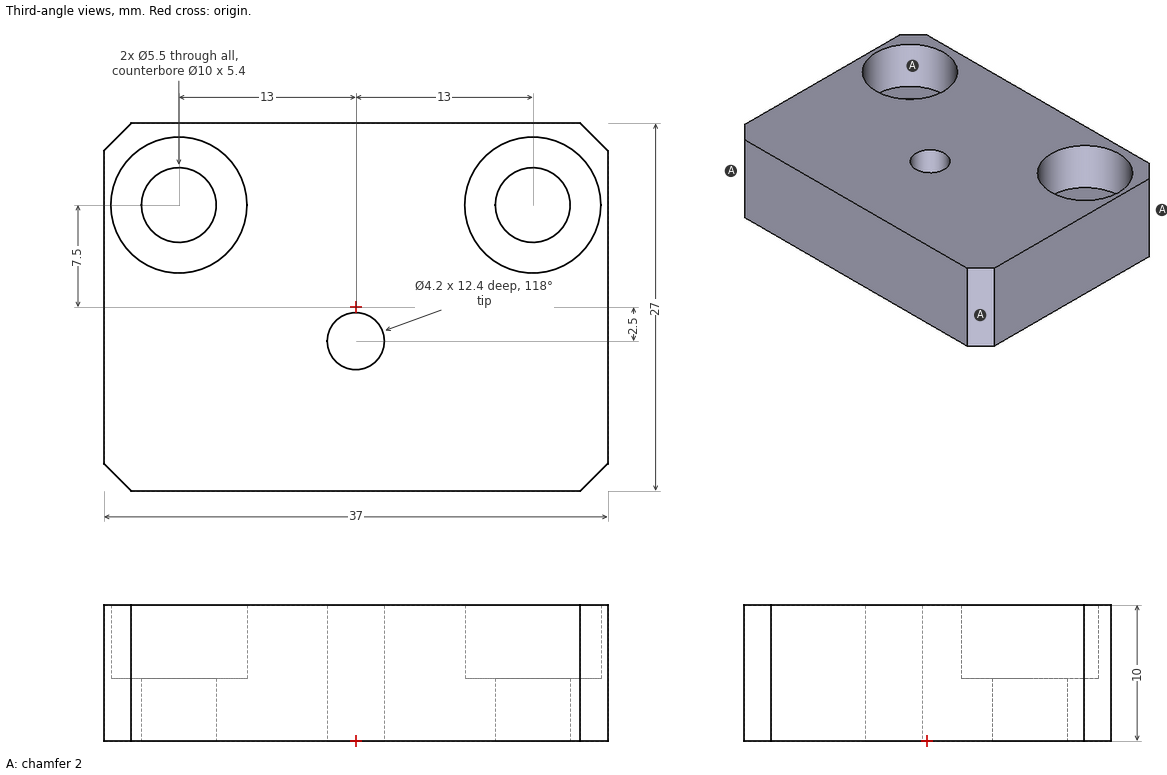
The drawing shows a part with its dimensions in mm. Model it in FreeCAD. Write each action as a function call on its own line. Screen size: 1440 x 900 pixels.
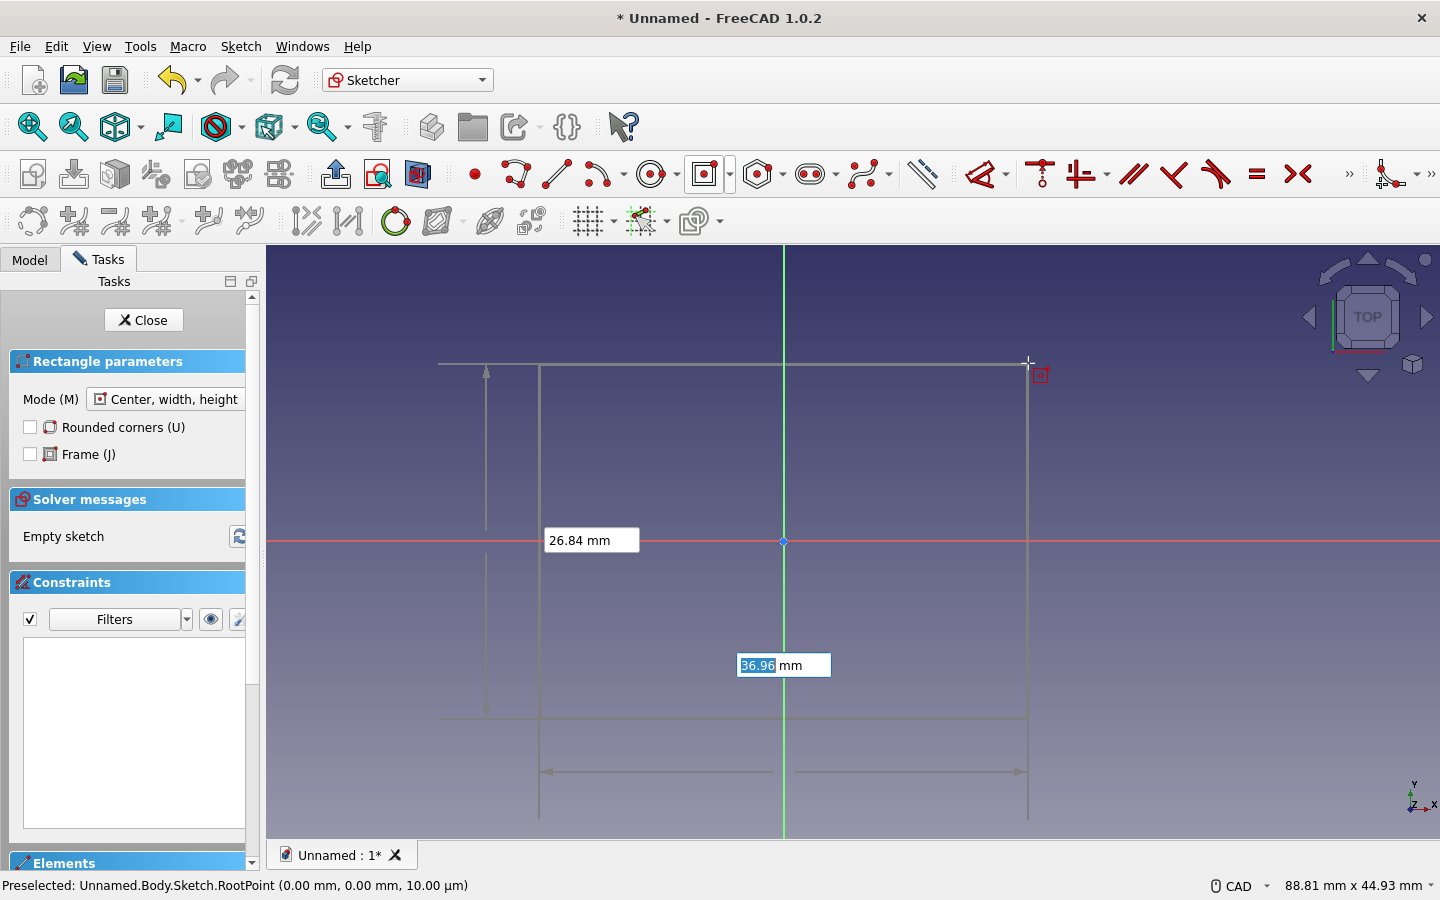
text(37)
key(Tab)
text(27)
key(Return)
key(Escape)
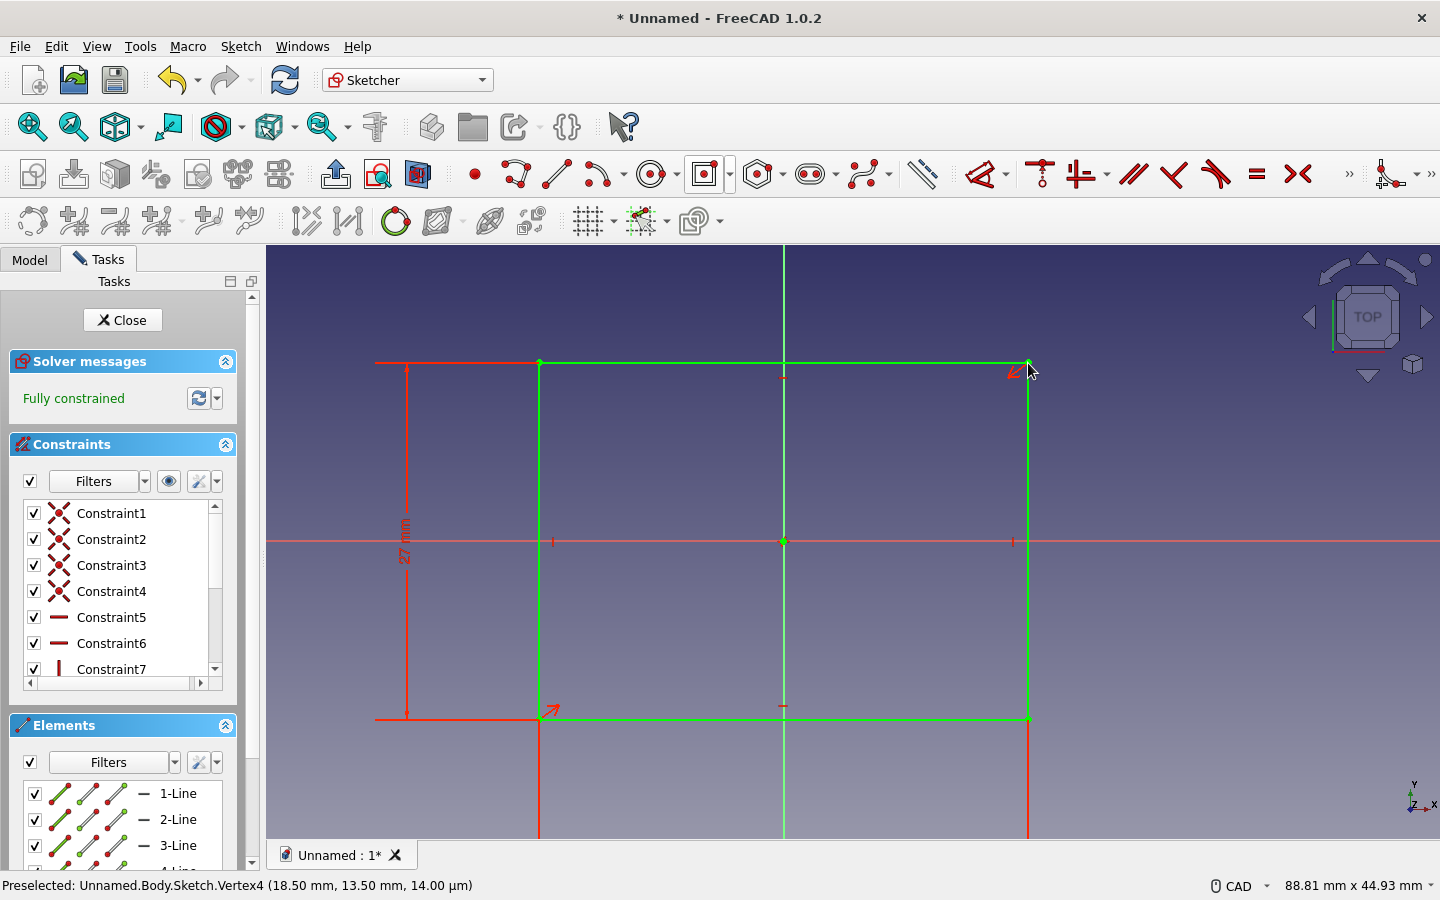
click(123, 320)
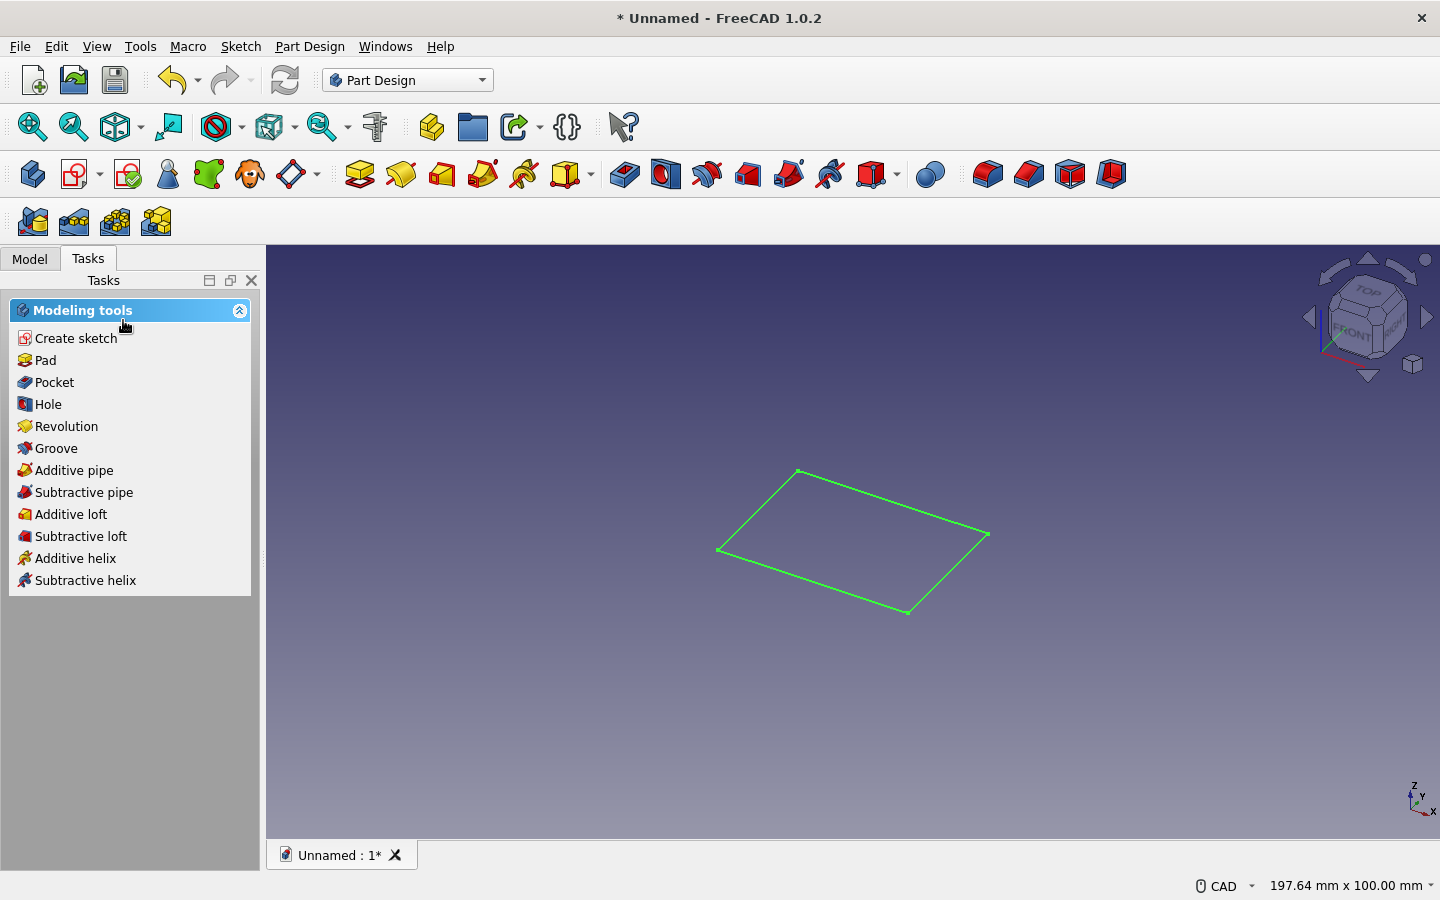
click(360, 174)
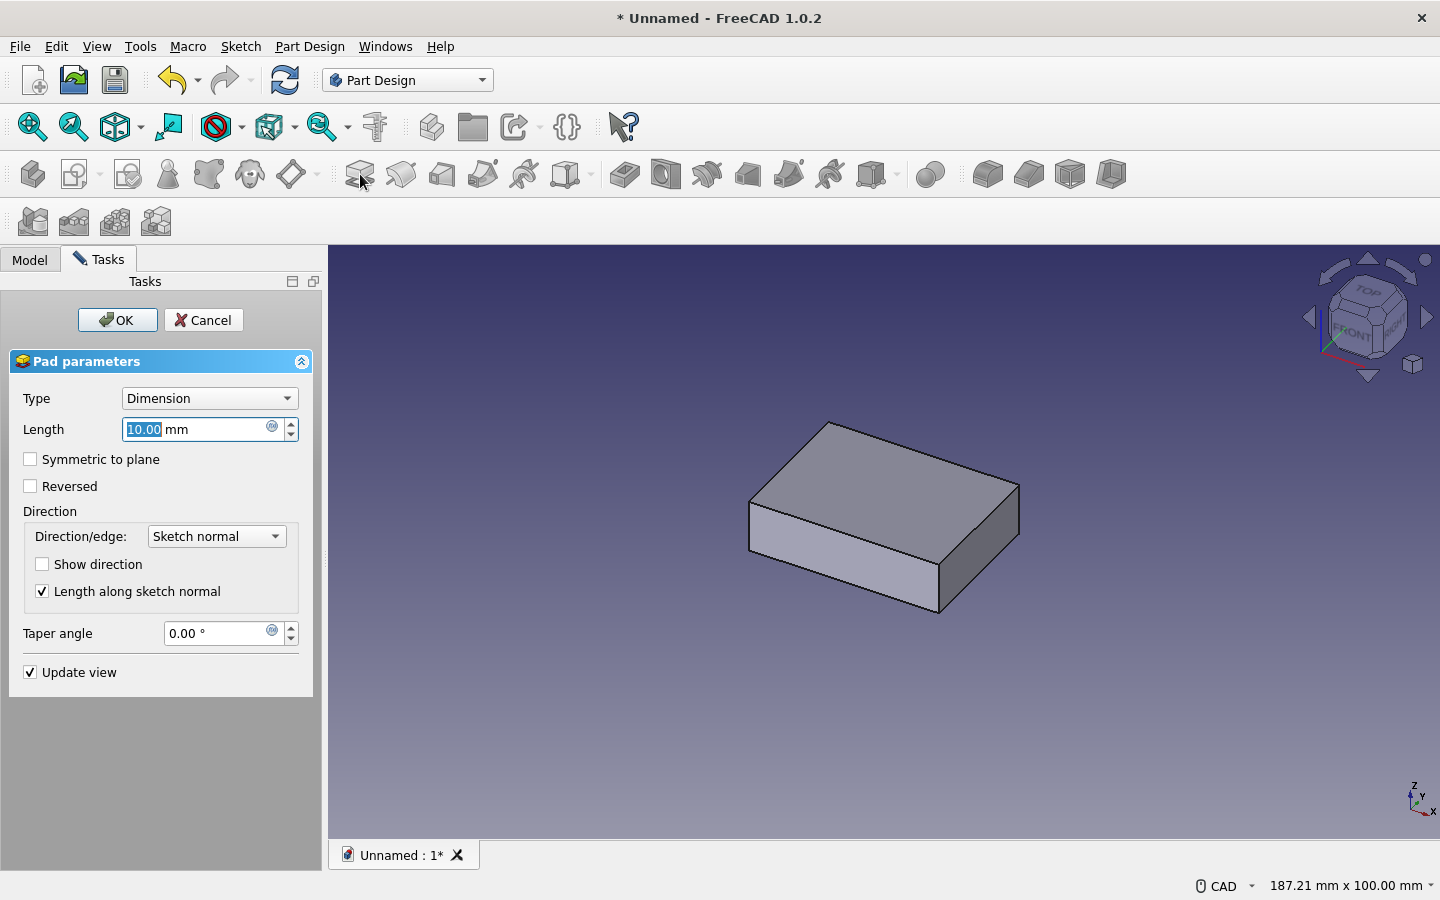
text(10)
key(Tab)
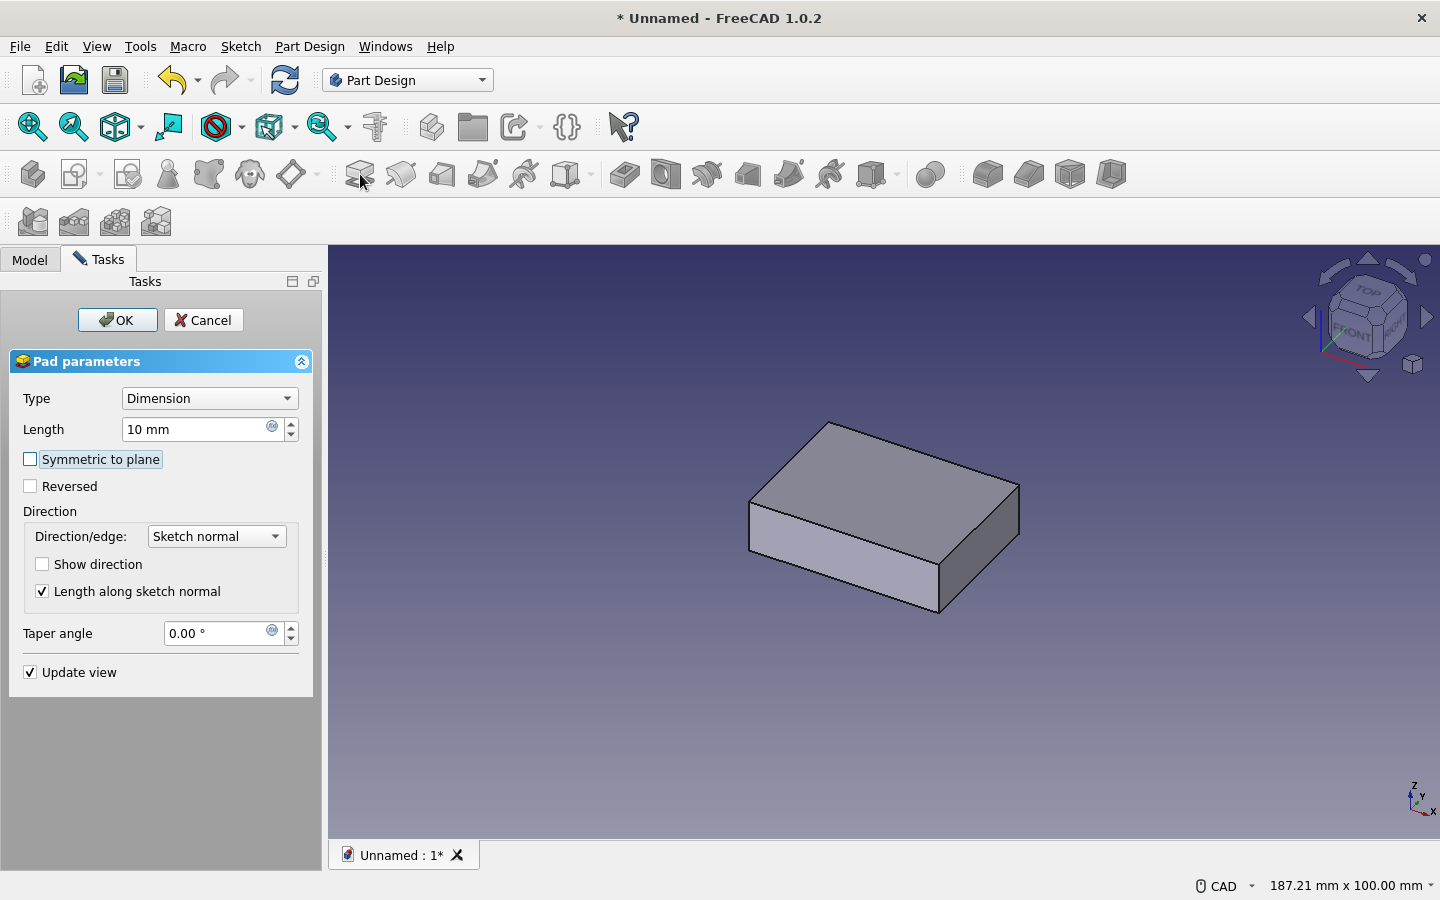
click(118, 320)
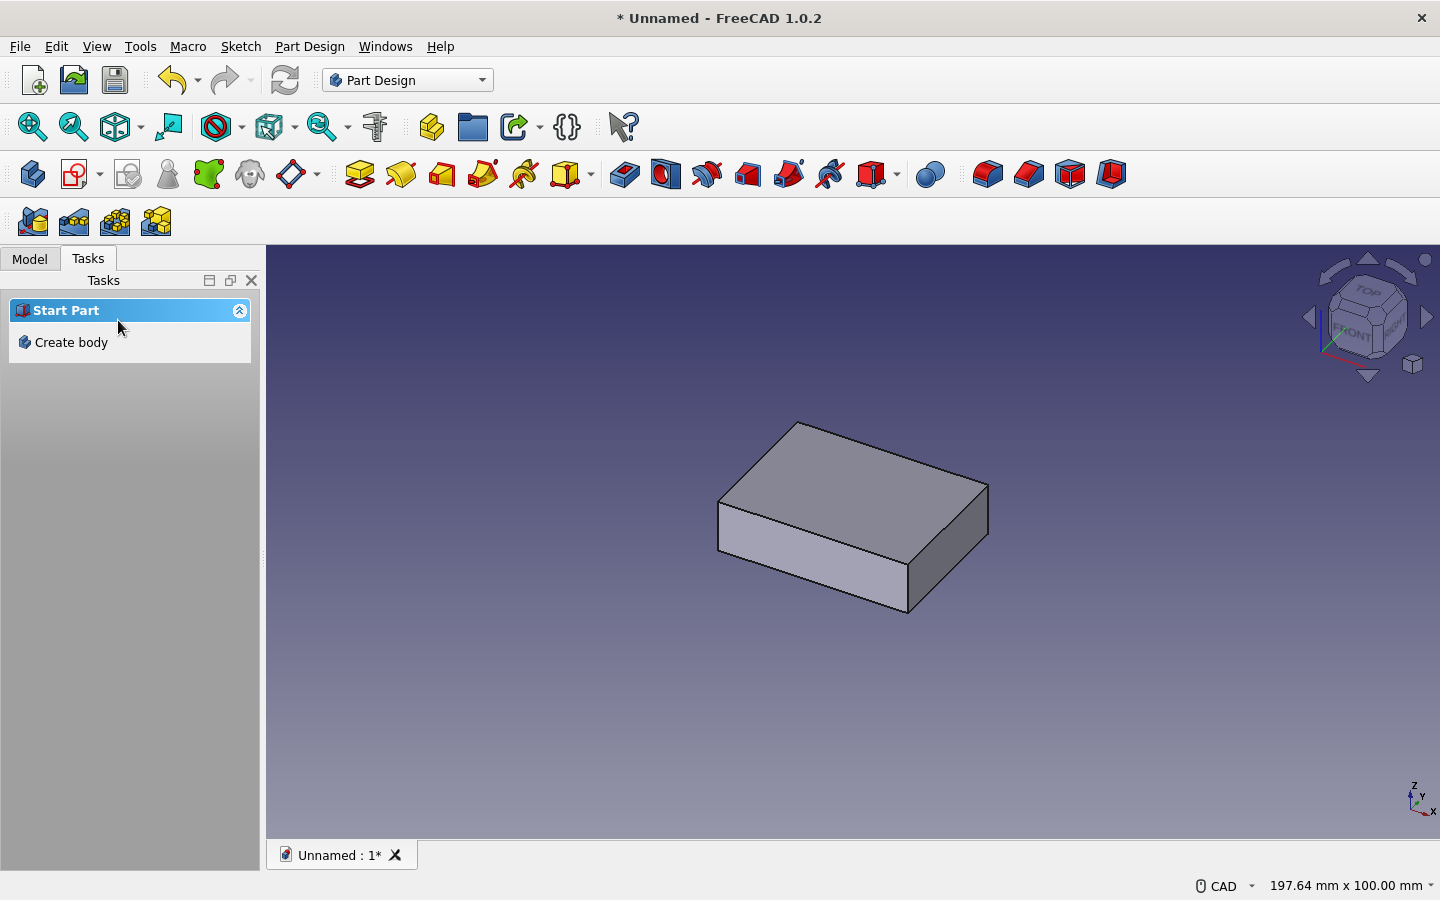
click(33, 128)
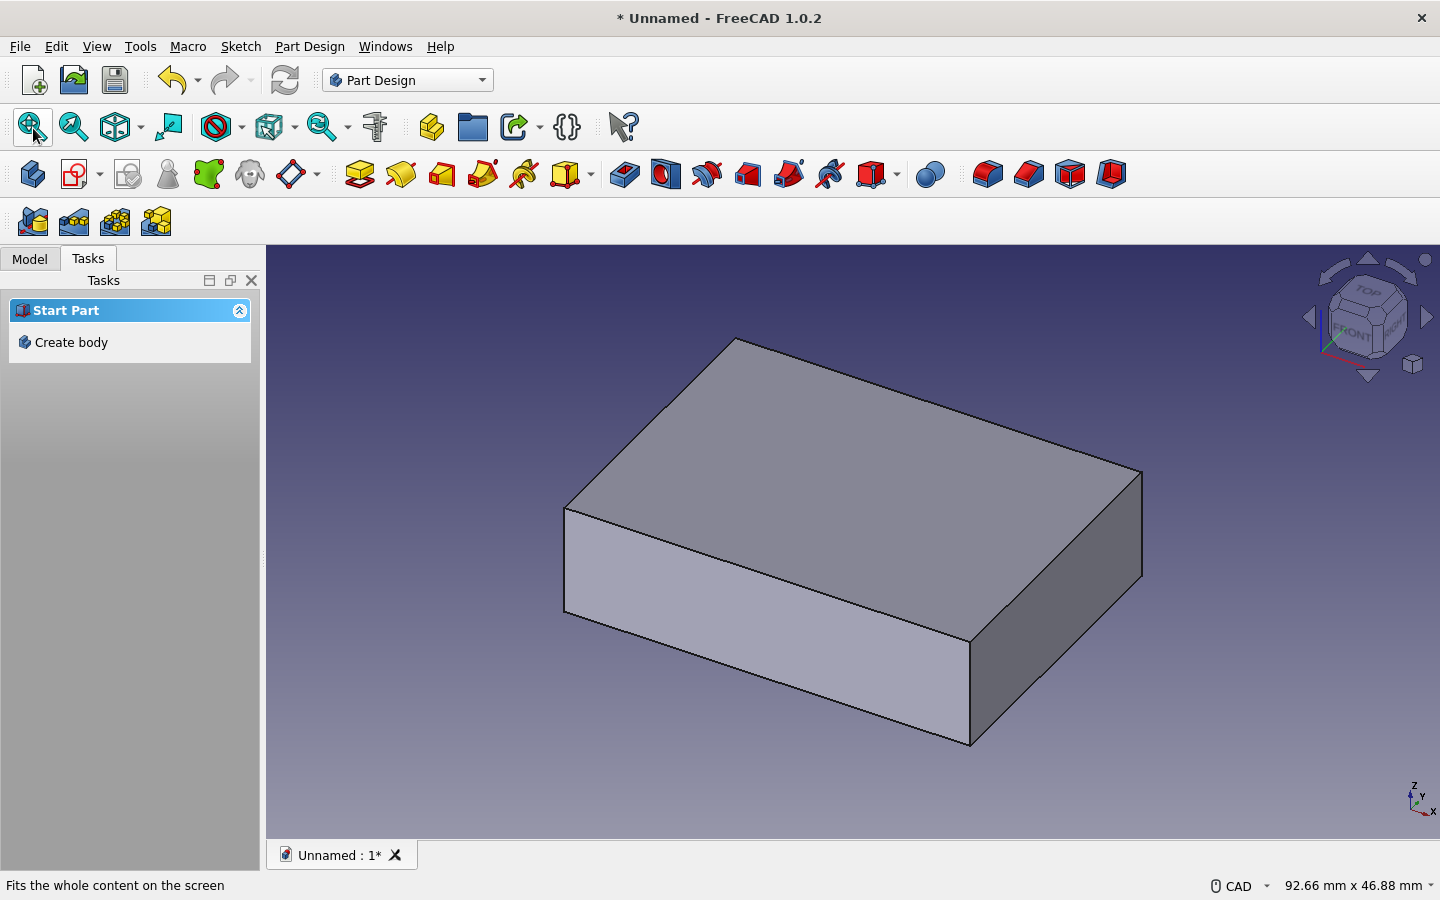
click(853, 489)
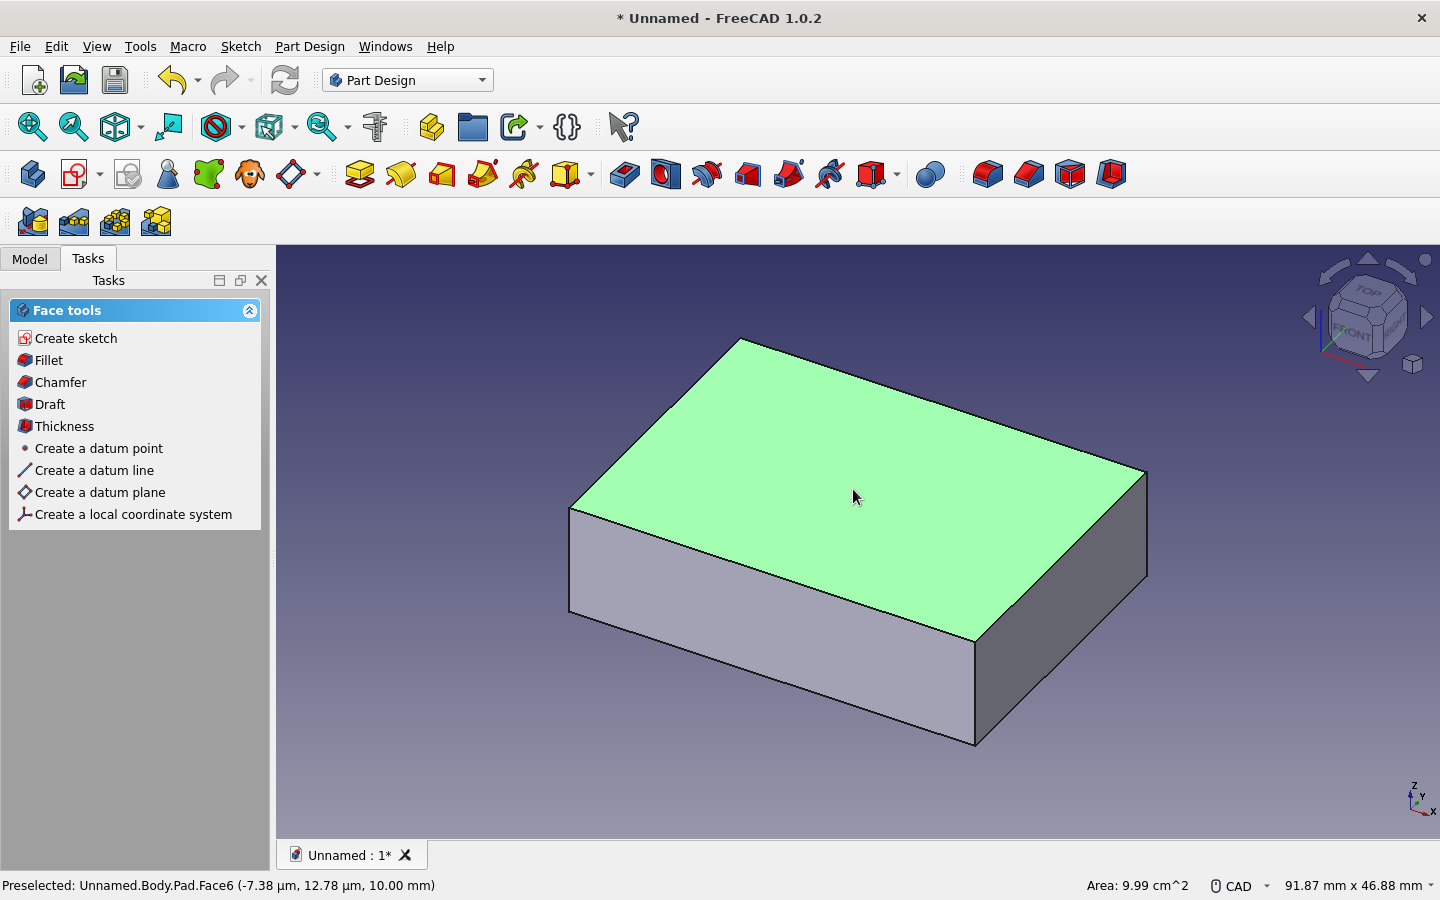
click(74, 174)